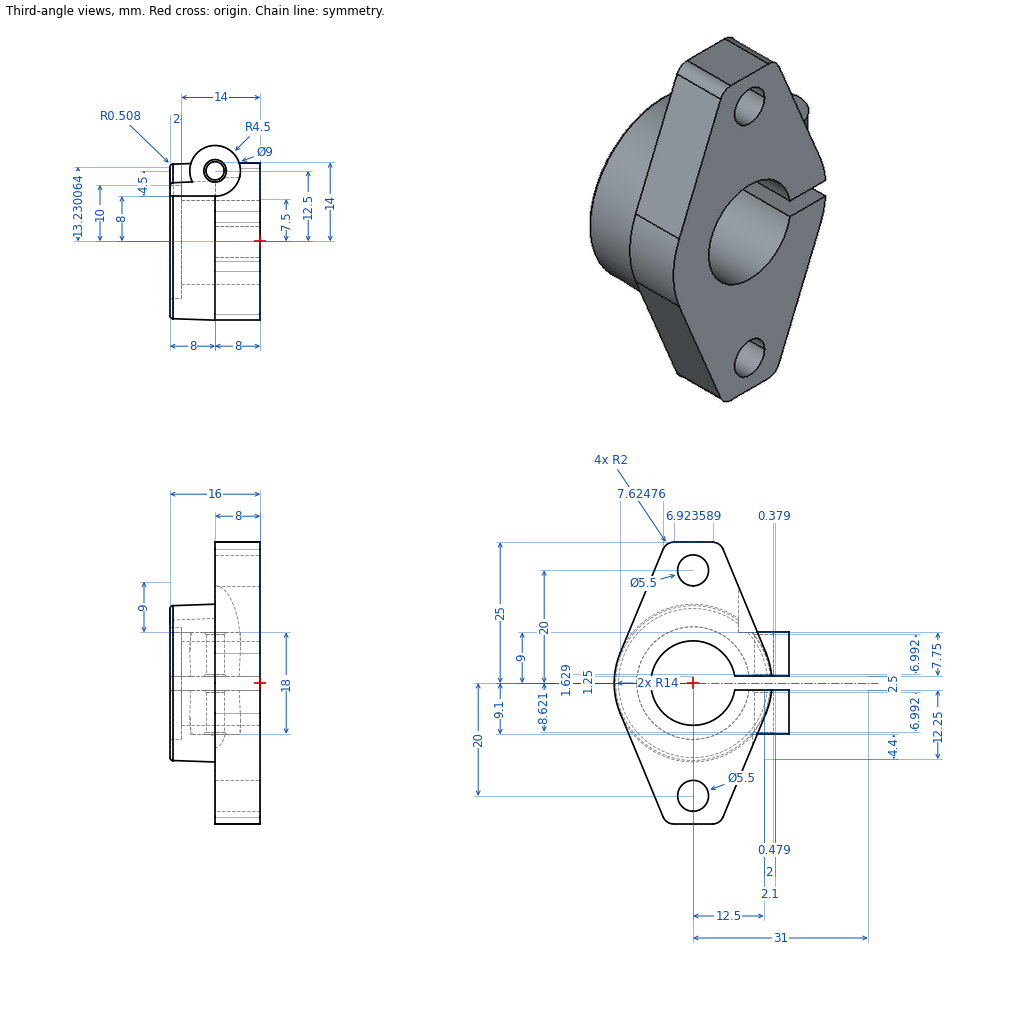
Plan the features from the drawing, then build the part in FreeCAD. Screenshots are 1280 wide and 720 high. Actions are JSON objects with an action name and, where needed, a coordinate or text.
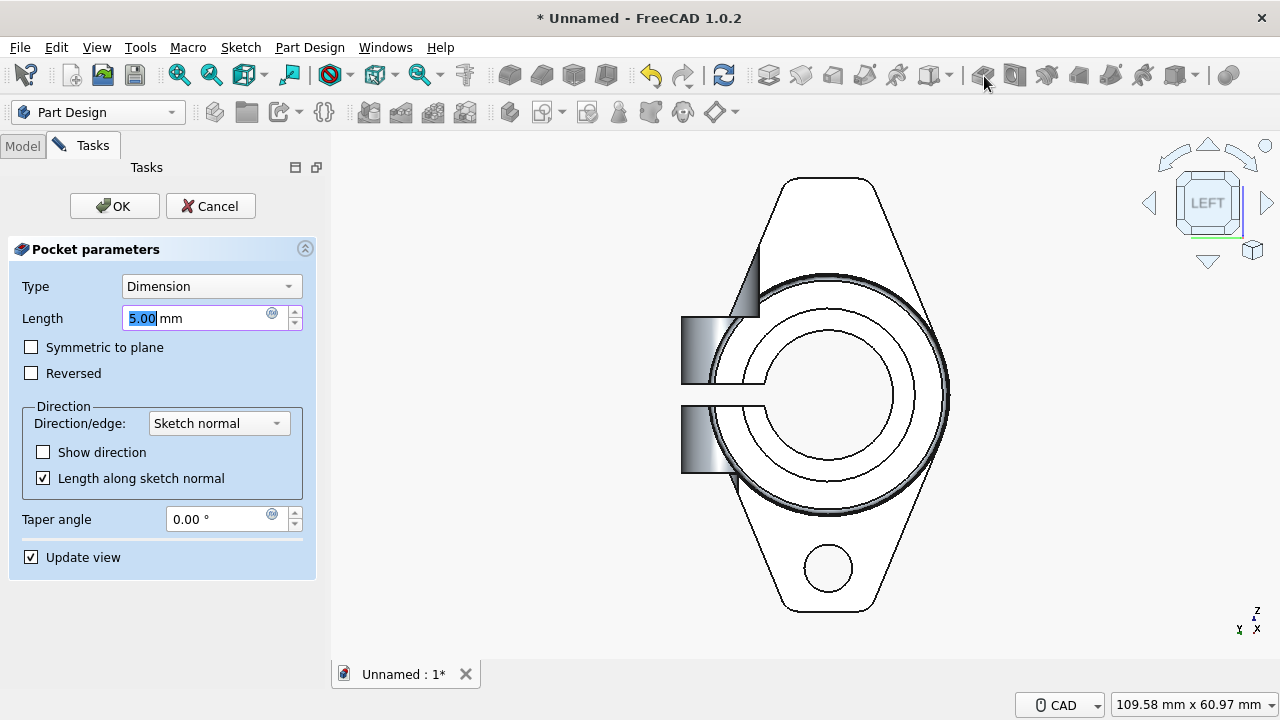
{"action": "type", "text": "8"}
{"action": "key", "text": "Tab"}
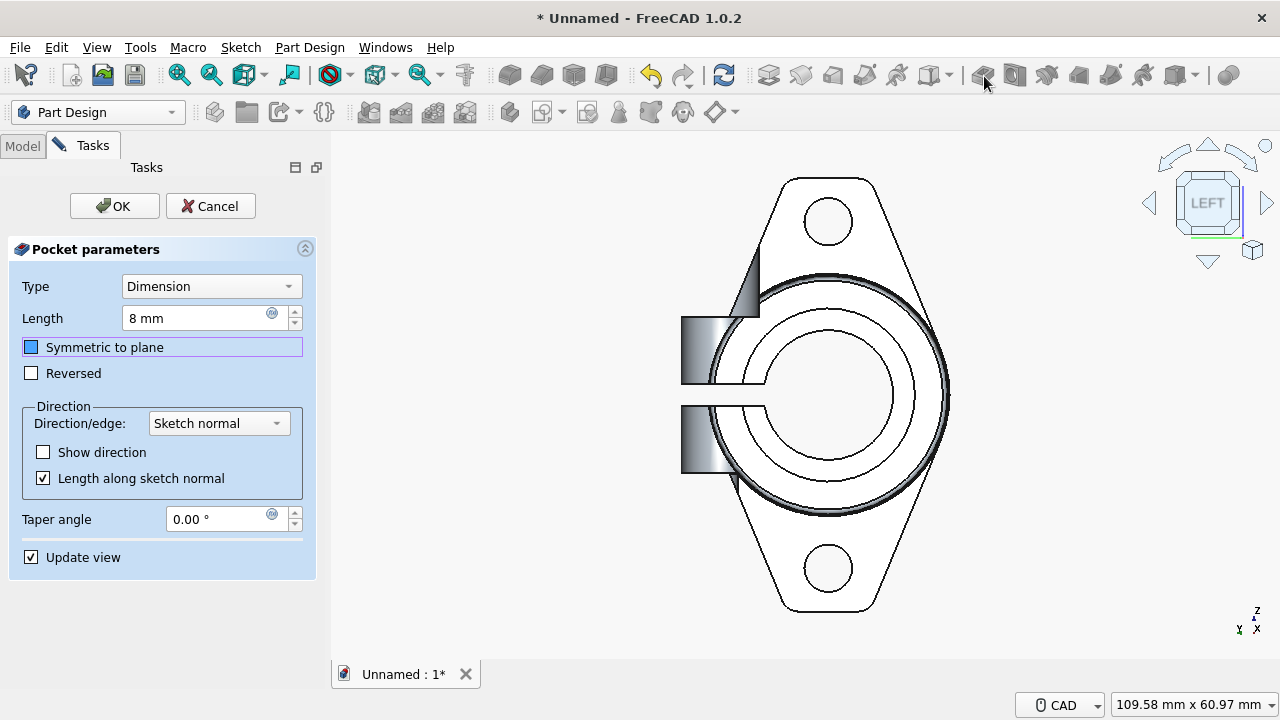
{"action": "left_click", "coordinate": [115, 206]}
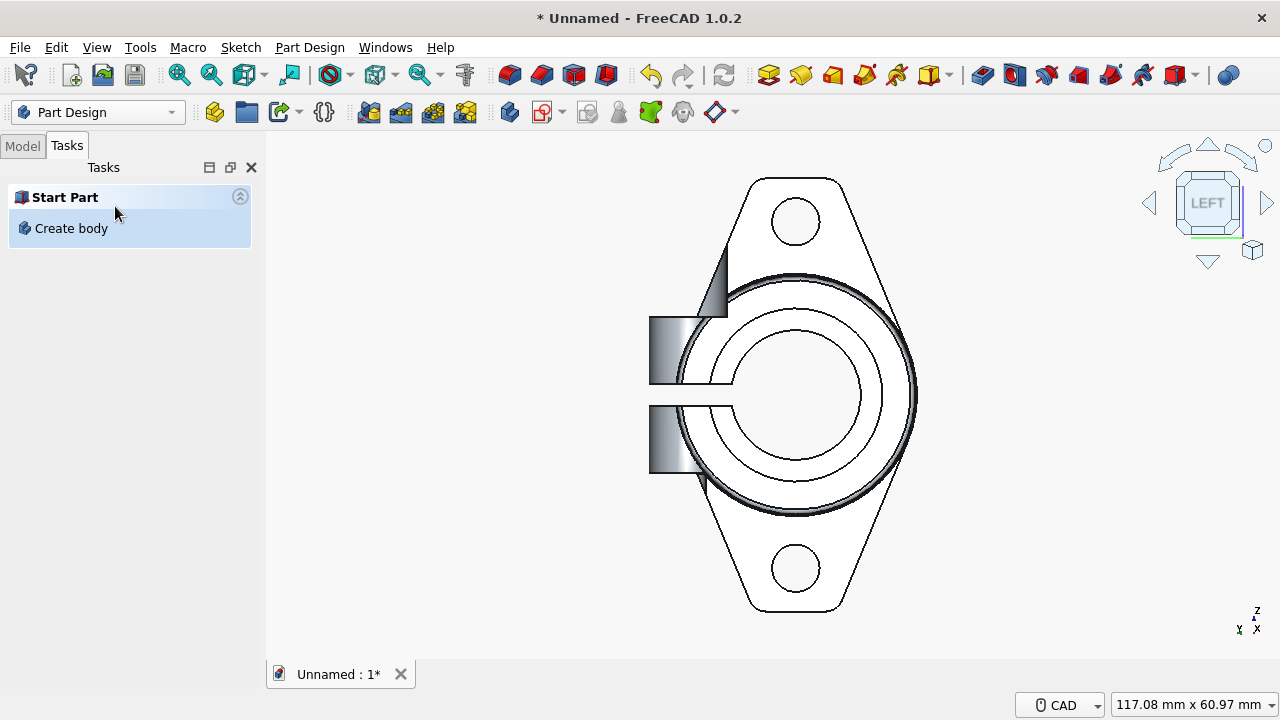
{"action": "key", "text": "0"}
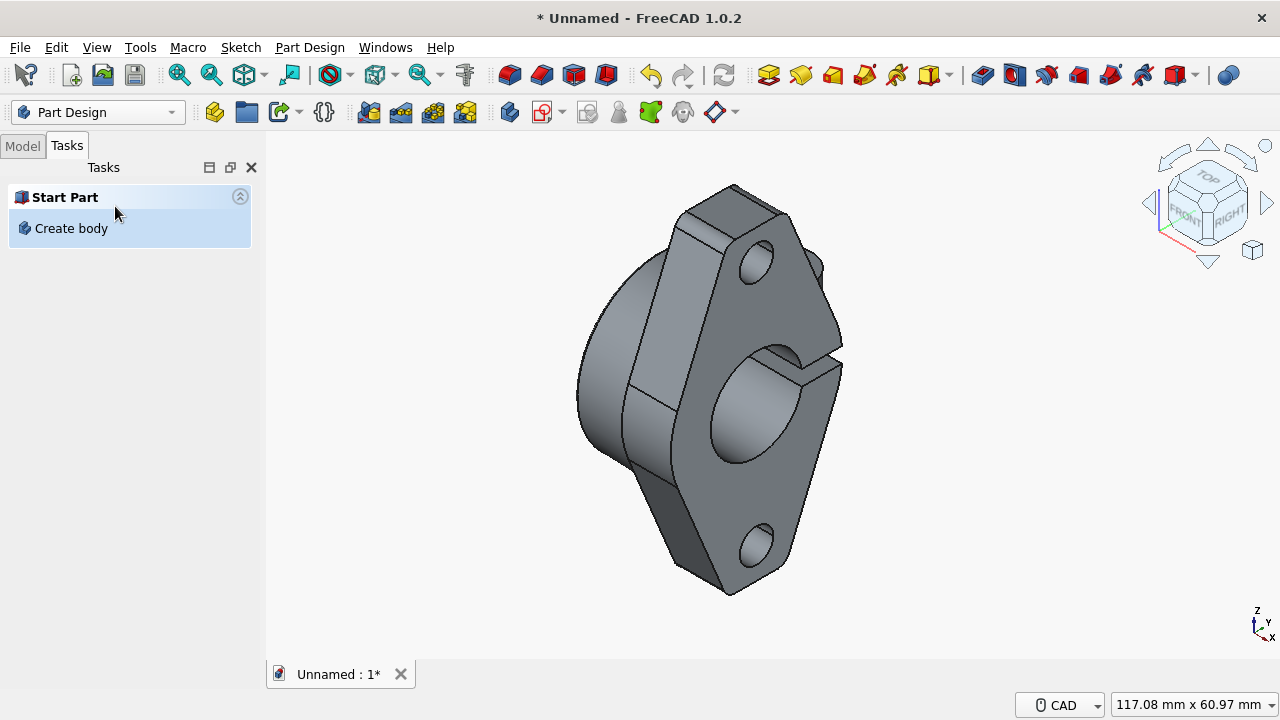
{"action": "left_click", "coordinate": [180, 76]}